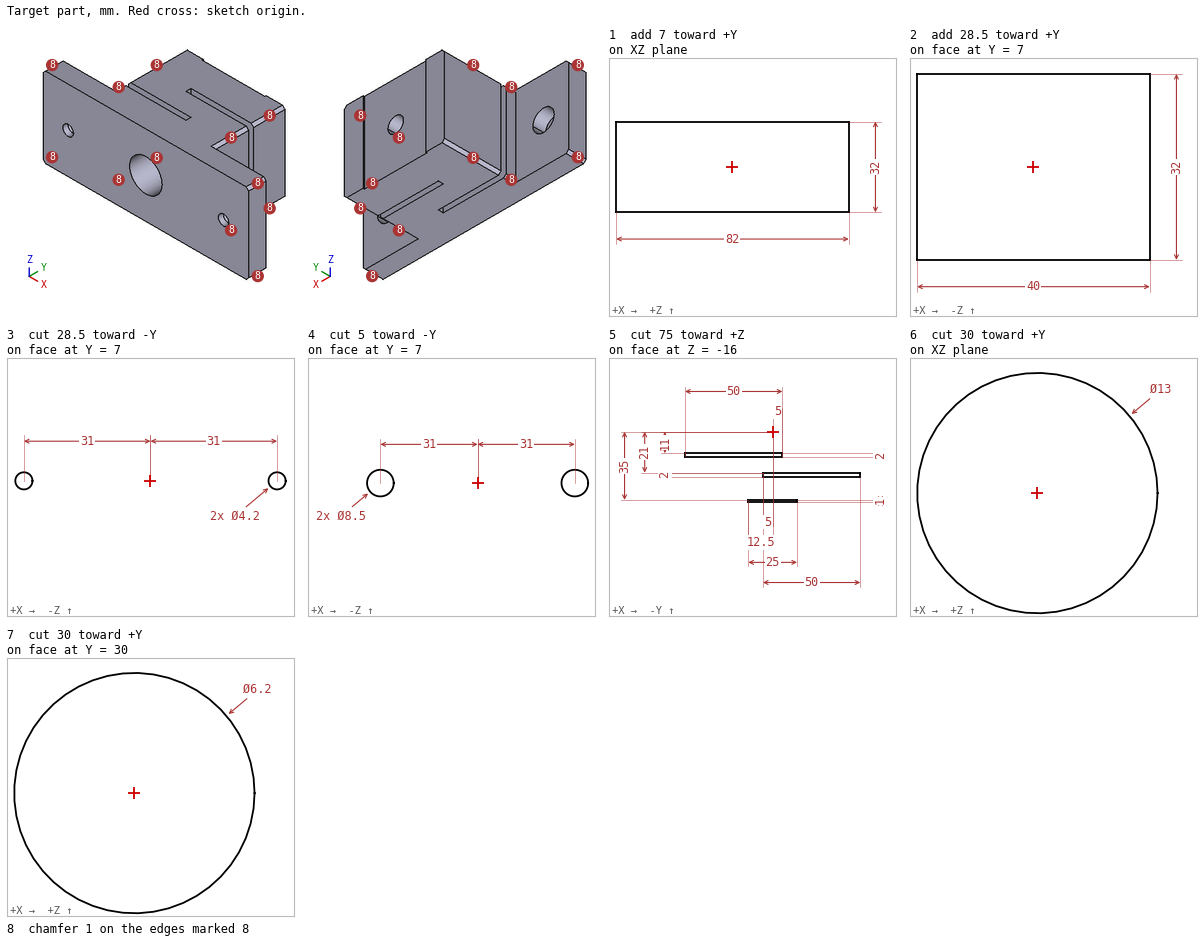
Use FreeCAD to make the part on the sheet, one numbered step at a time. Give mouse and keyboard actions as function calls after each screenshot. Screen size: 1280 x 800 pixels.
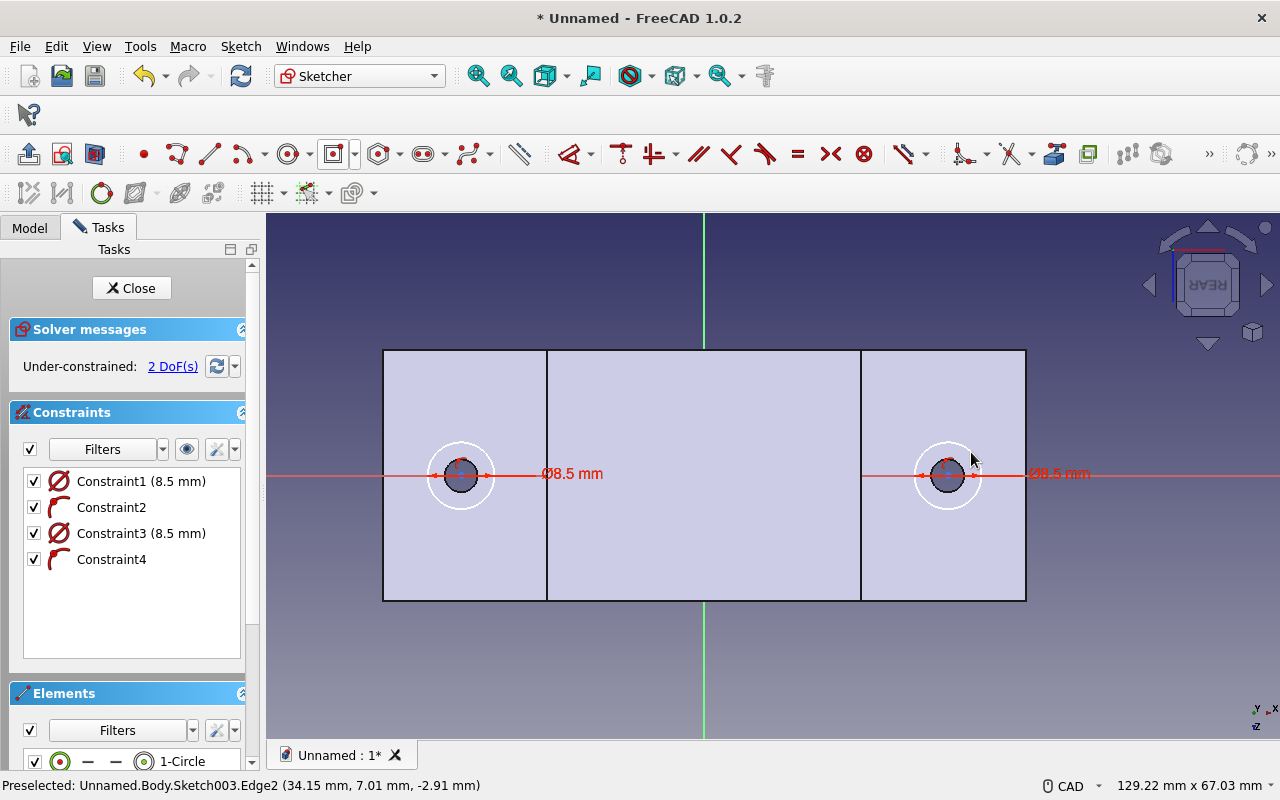
click(568, 154)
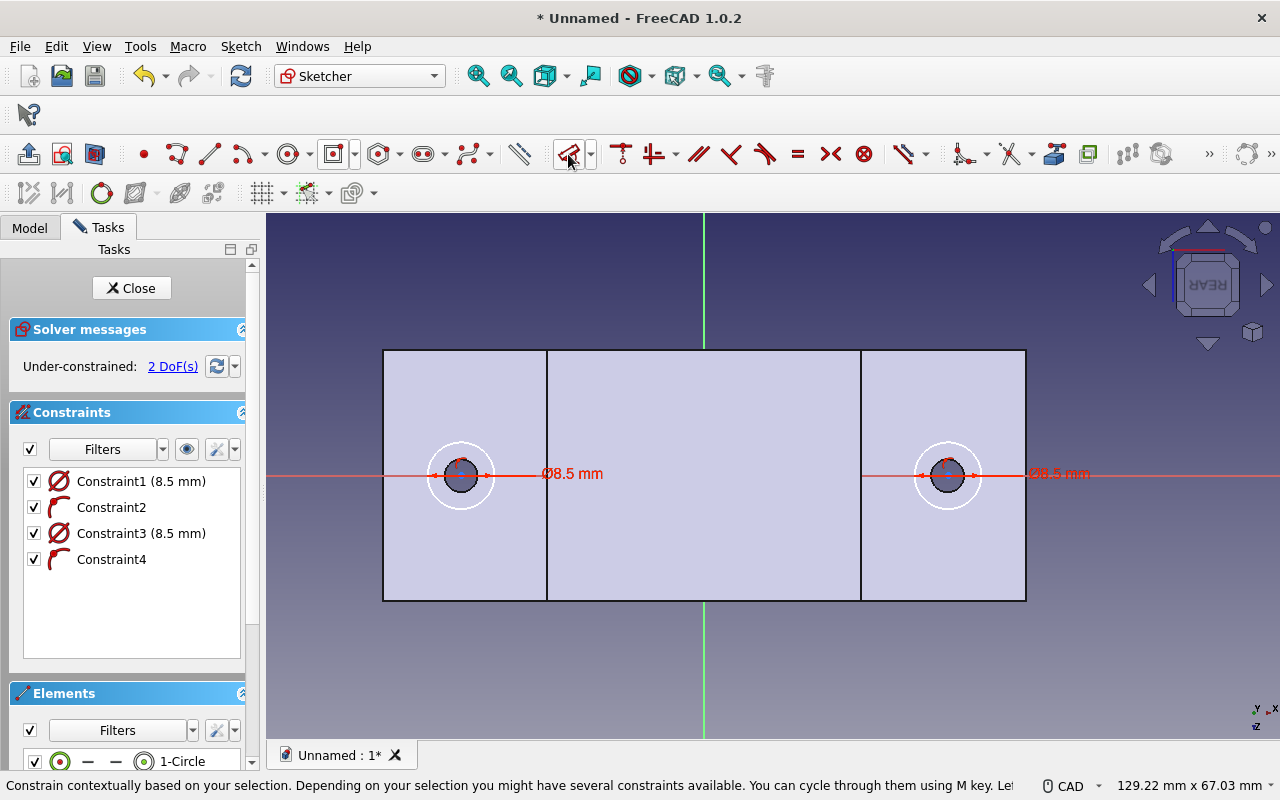
click(461, 476)
click(583, 510)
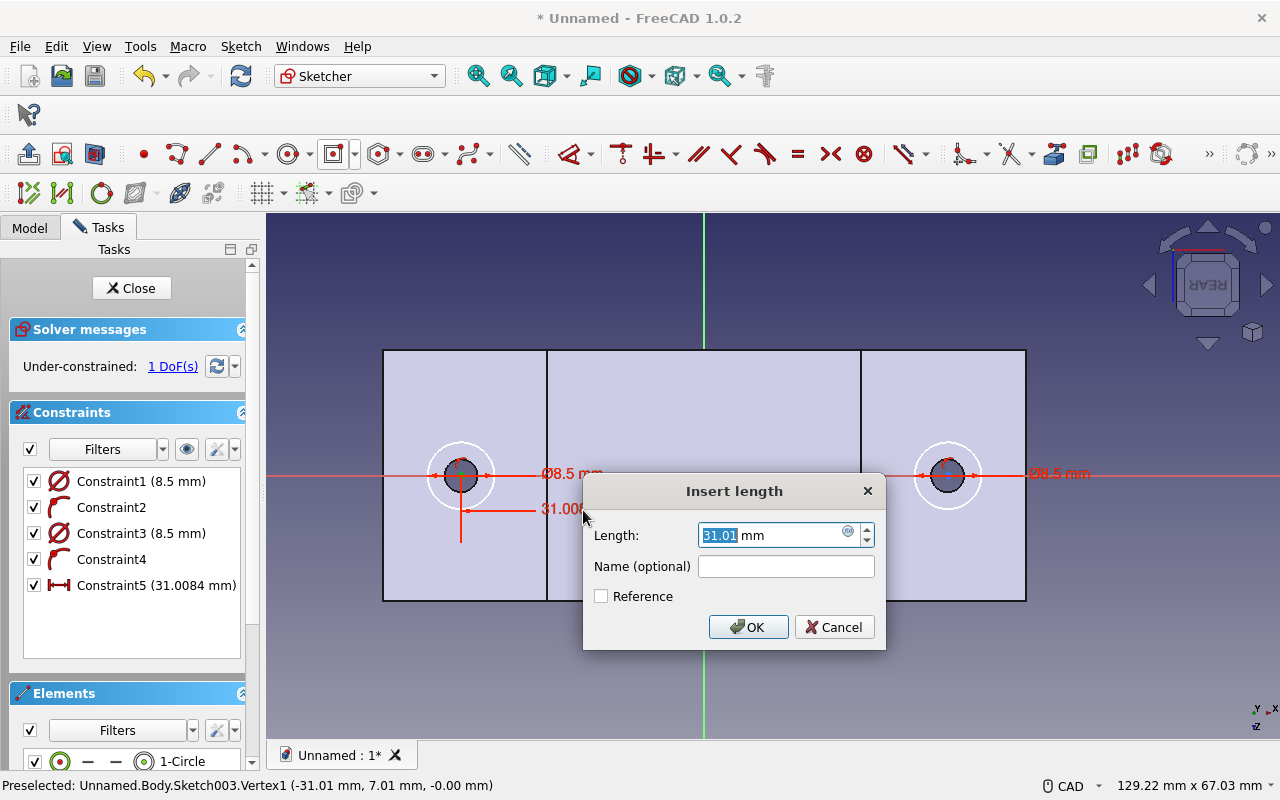
text(31)
key(Return)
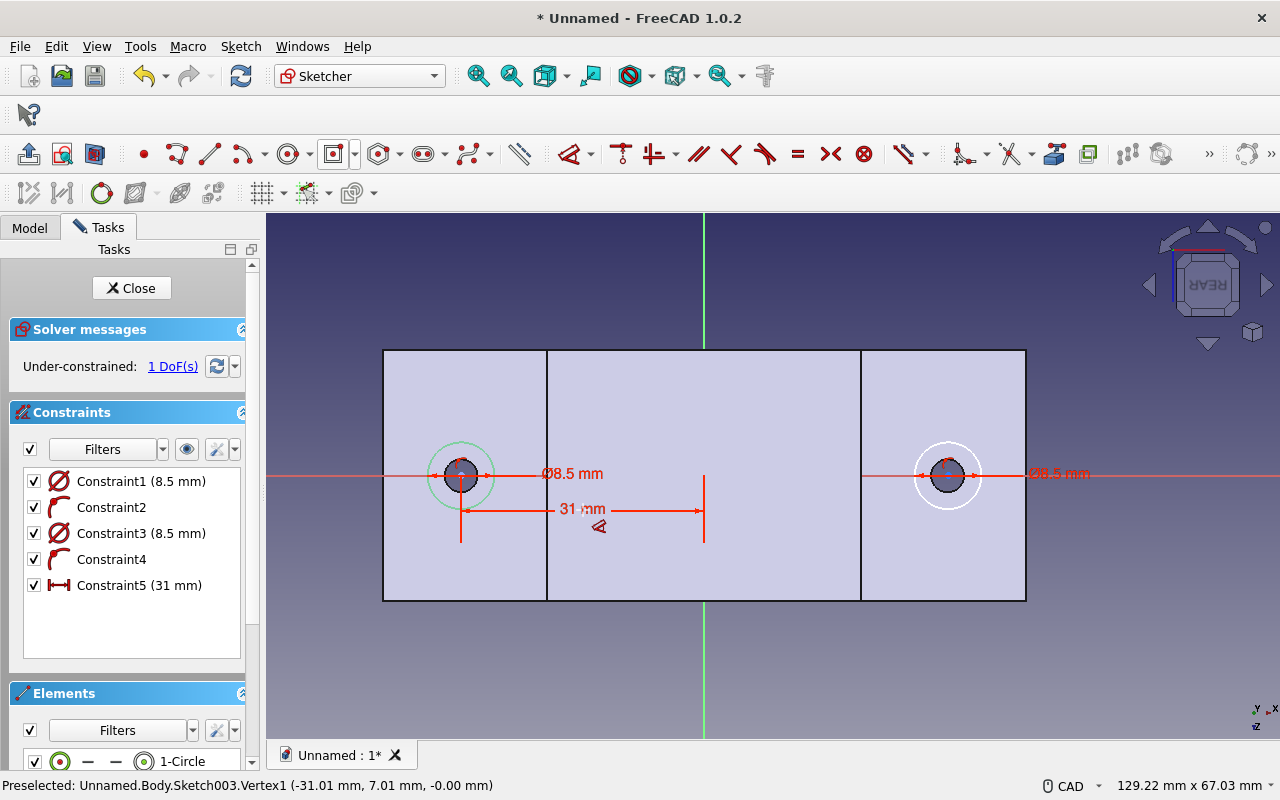
click(948, 476)
click(826, 510)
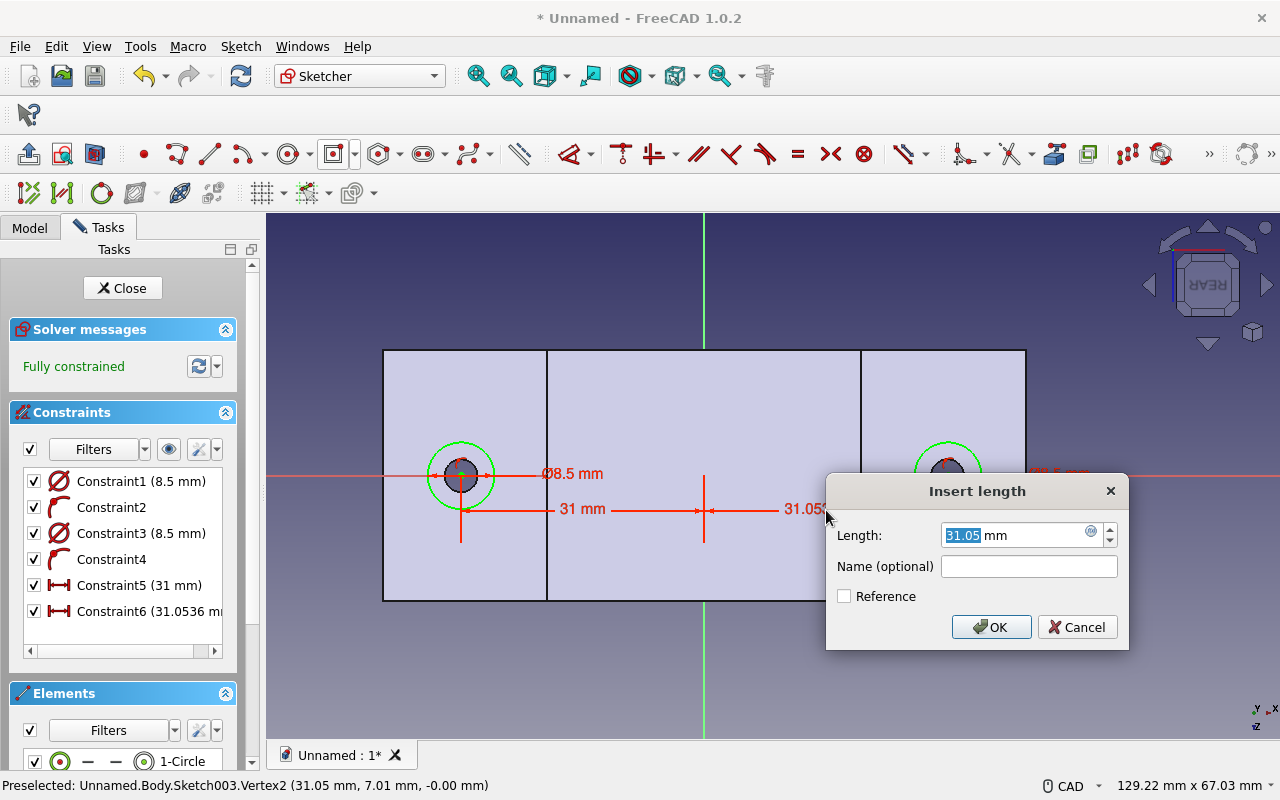
text(31)
key(Return)
key(Escape)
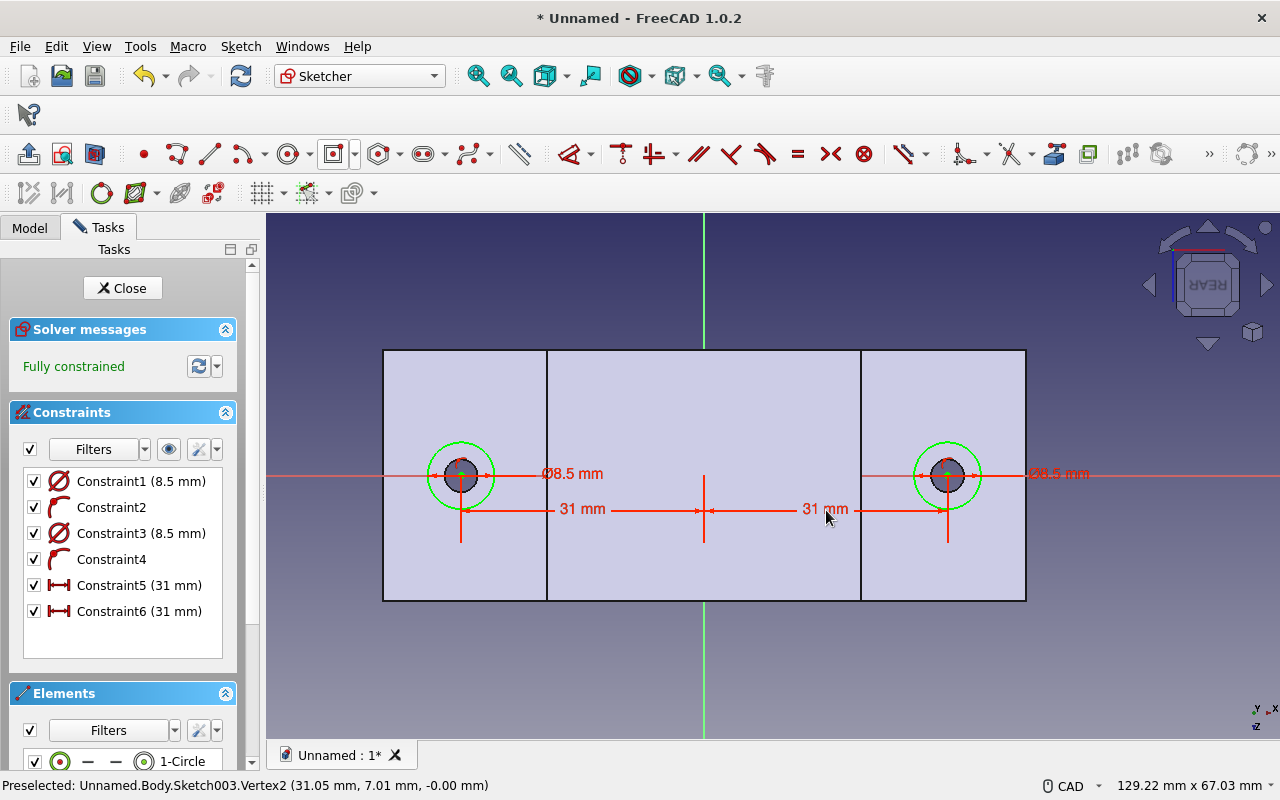
click(123, 288)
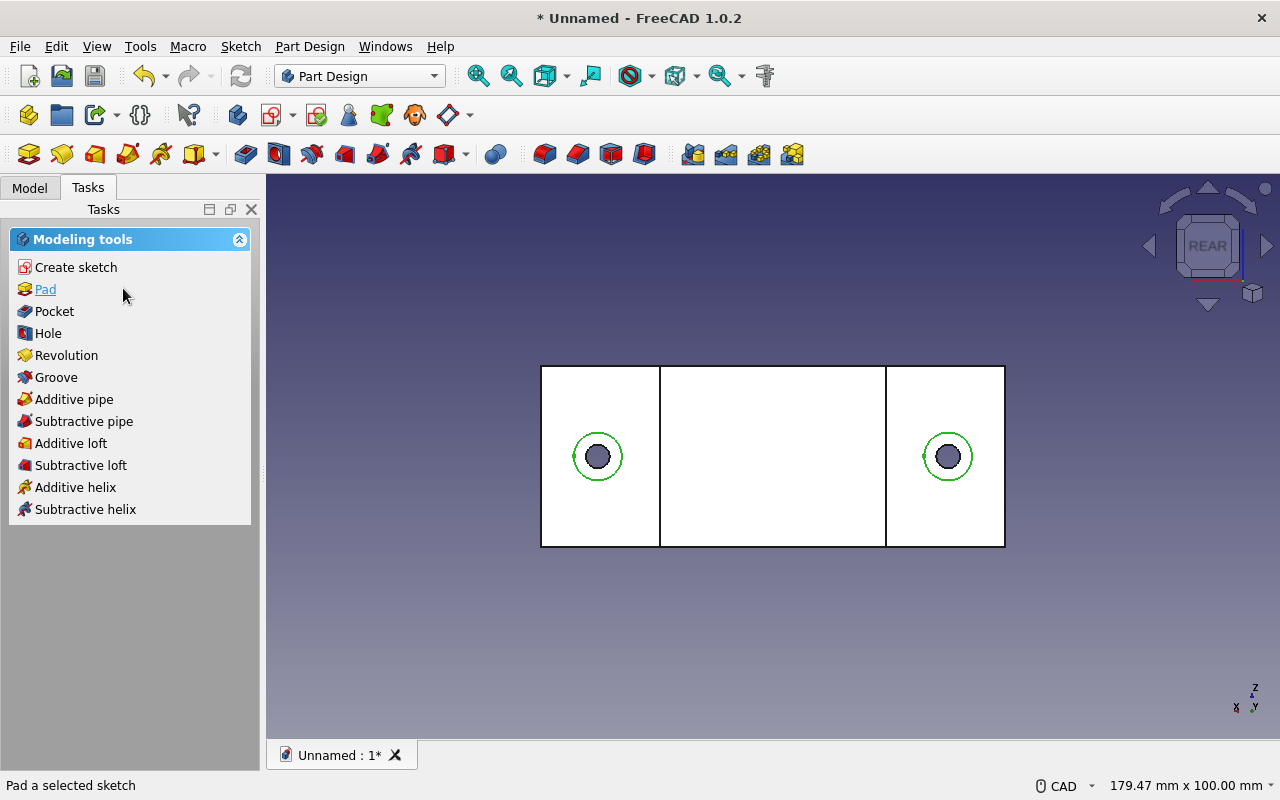
click(246, 154)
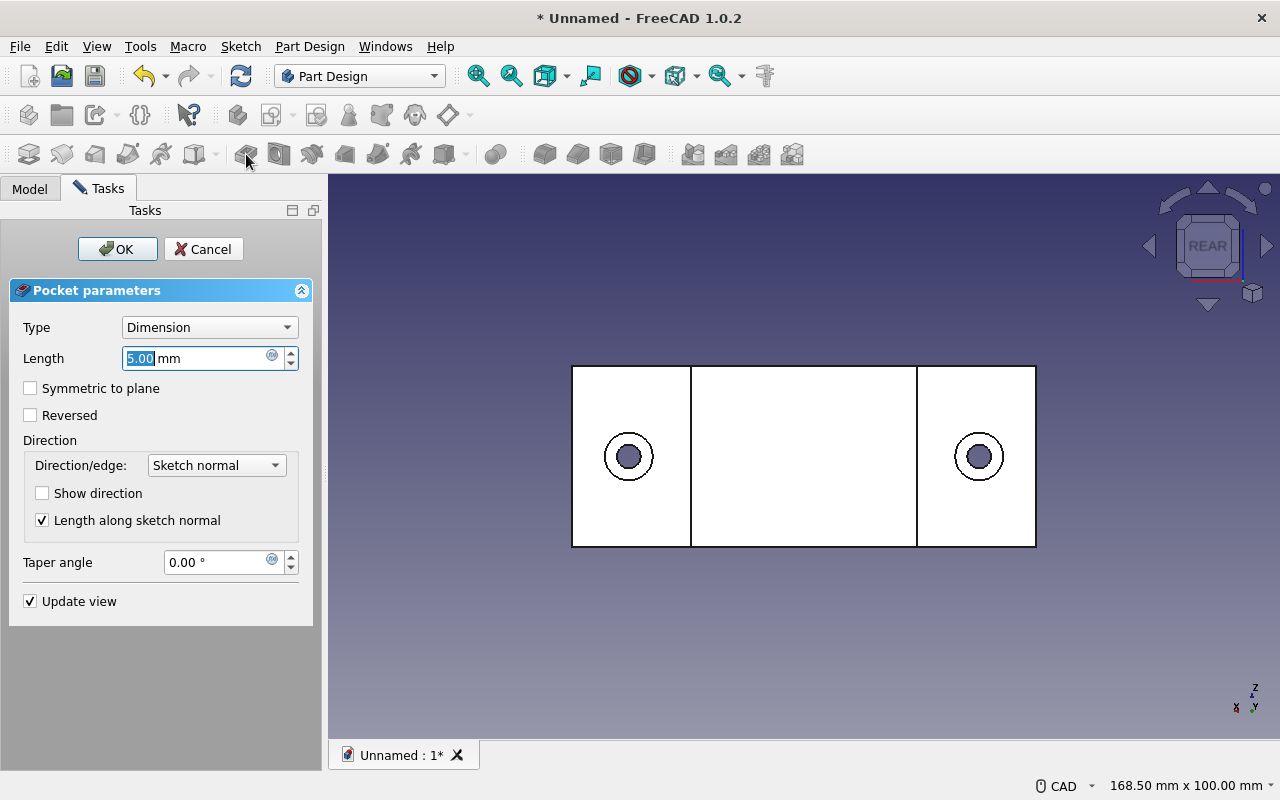
text(5)
key(Tab)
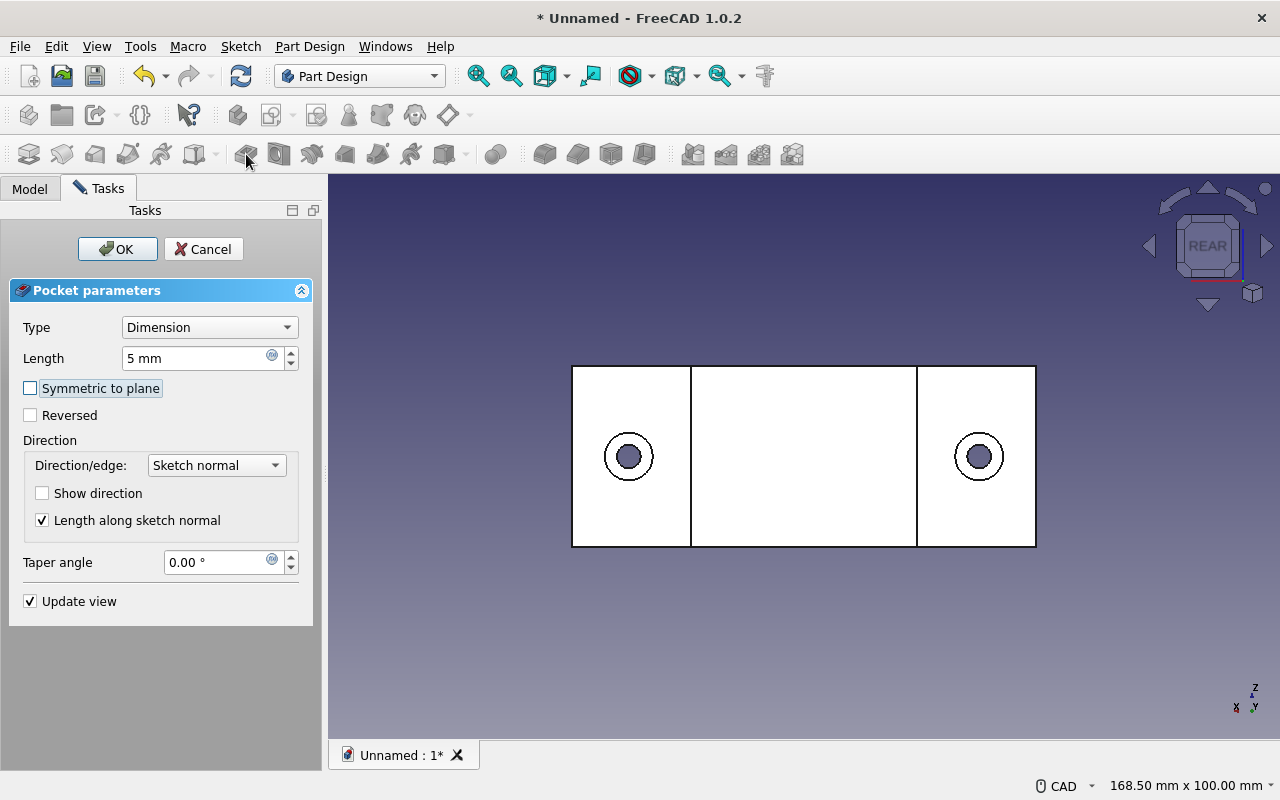
click(118, 249)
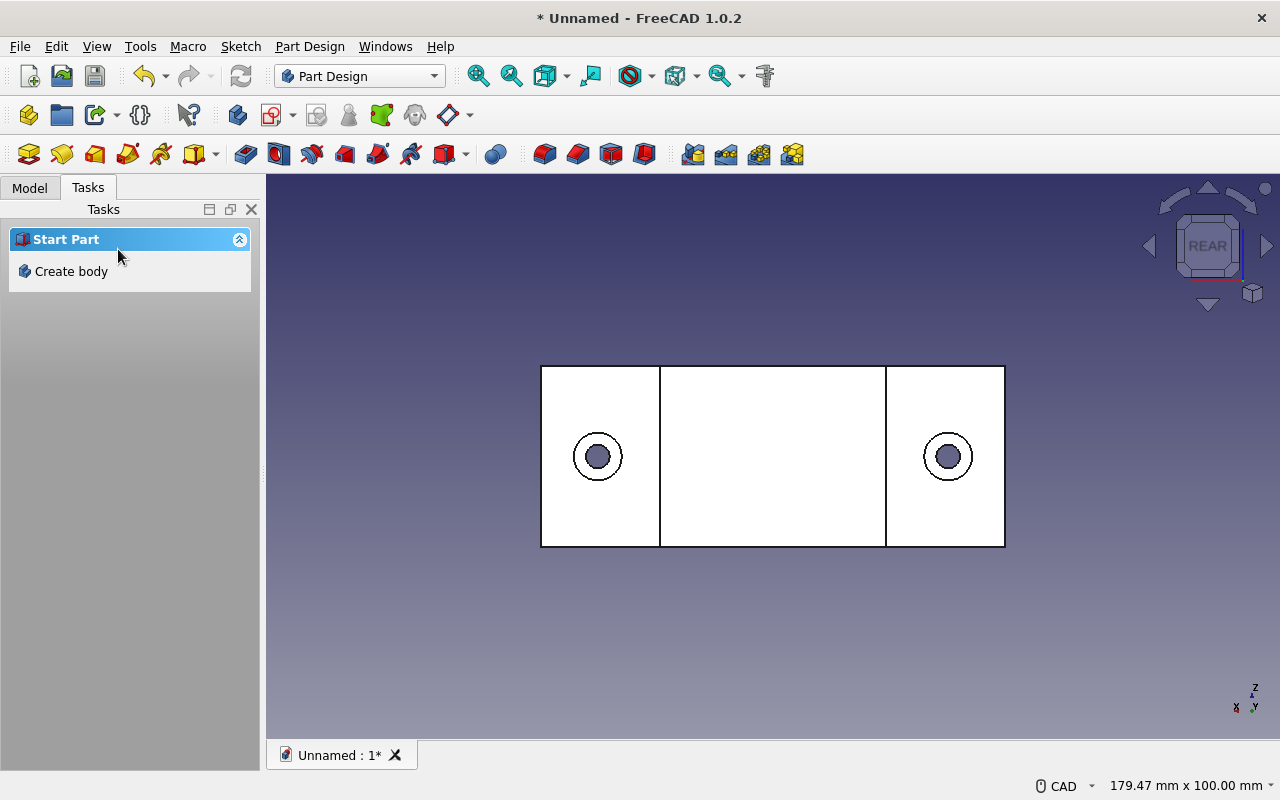
key(5)